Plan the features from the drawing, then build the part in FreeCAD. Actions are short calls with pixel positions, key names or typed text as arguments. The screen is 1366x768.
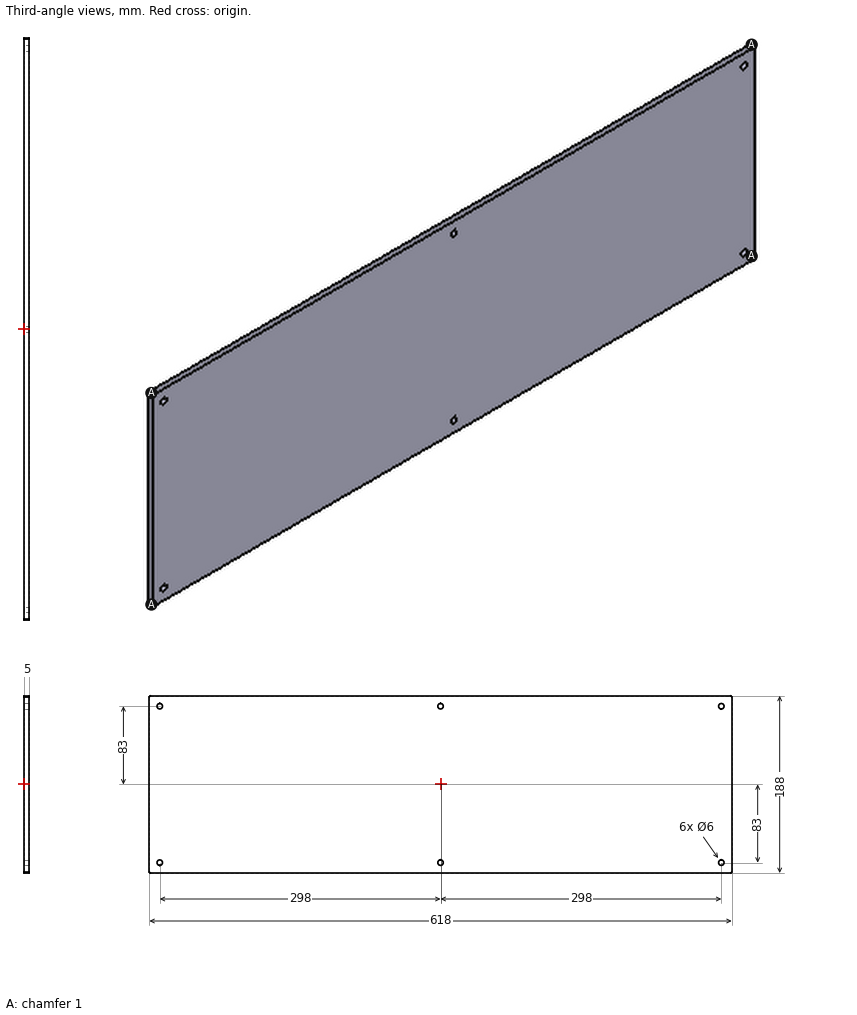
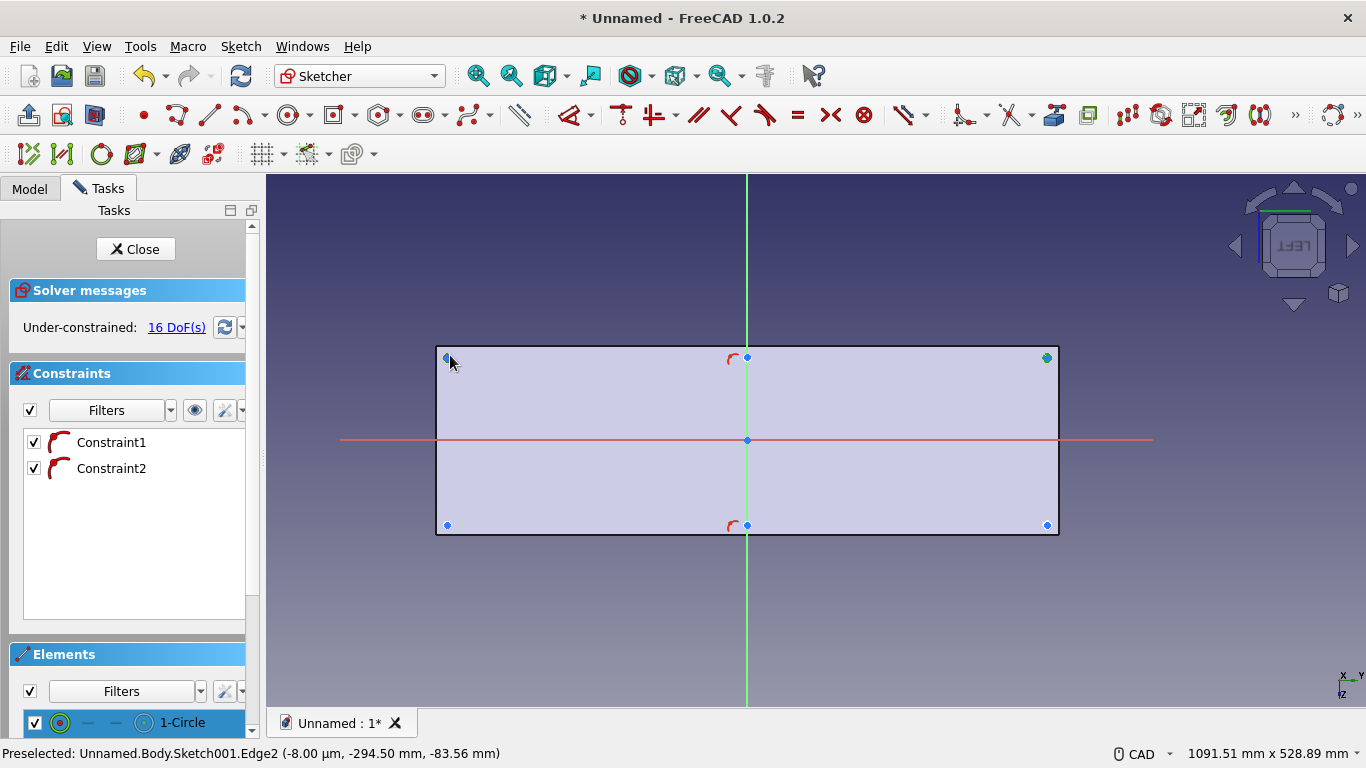
scroll(450, 523, up, 7)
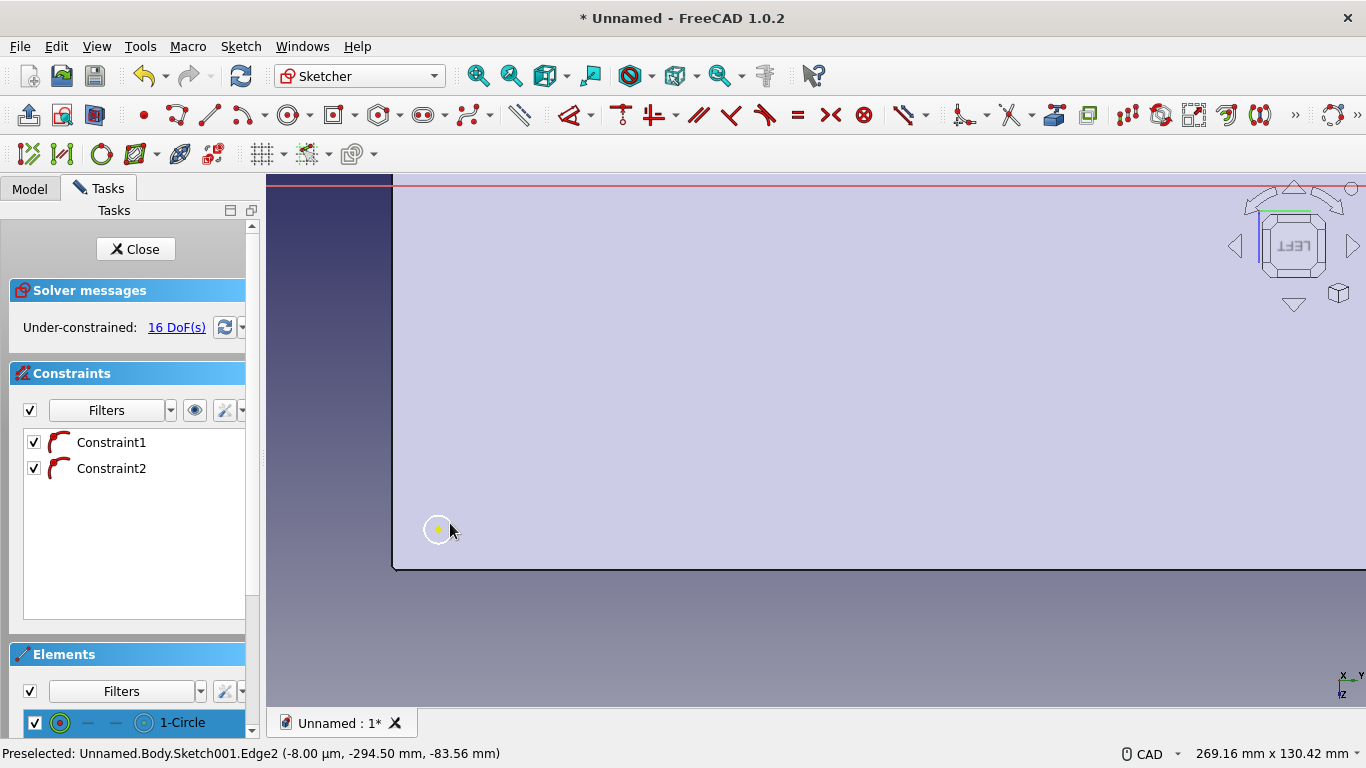
click(448, 520)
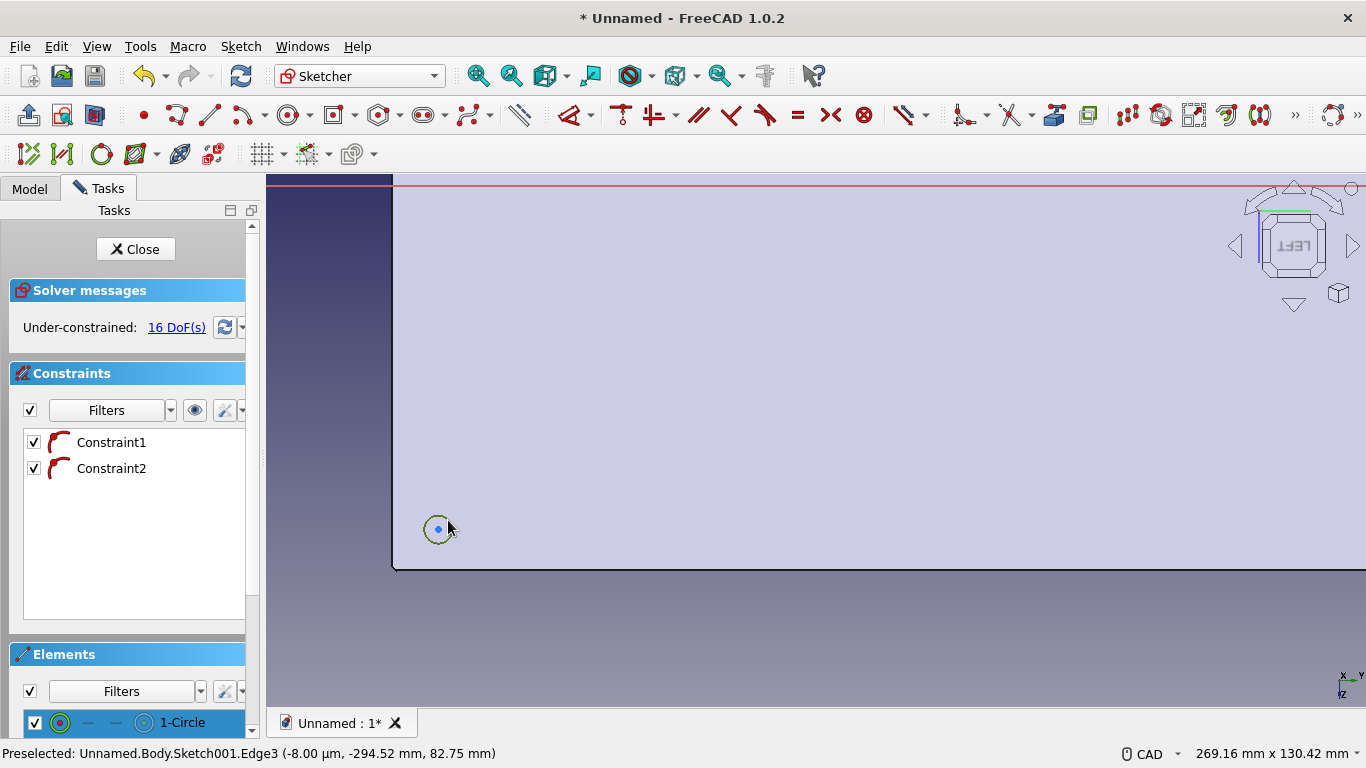
scroll(450, 524, down, 7)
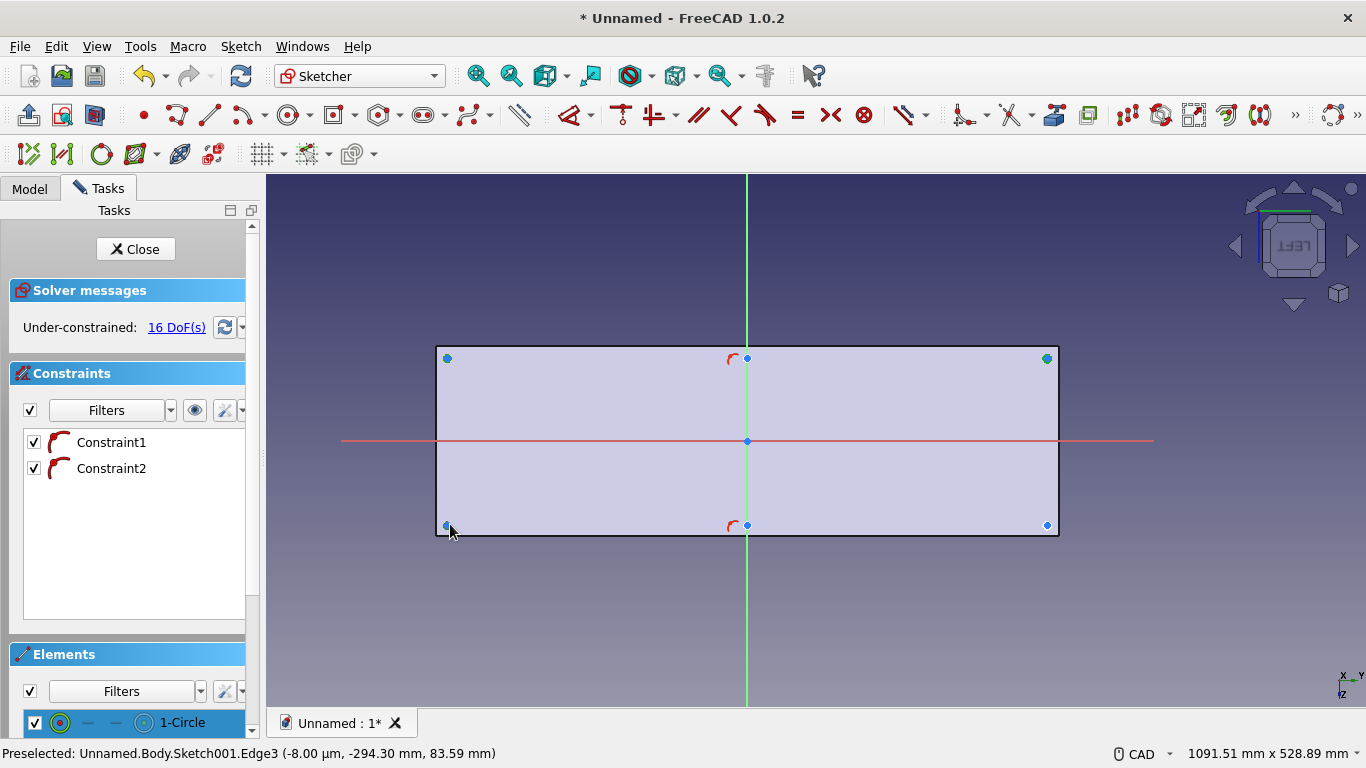
scroll(1050, 523, up, 7)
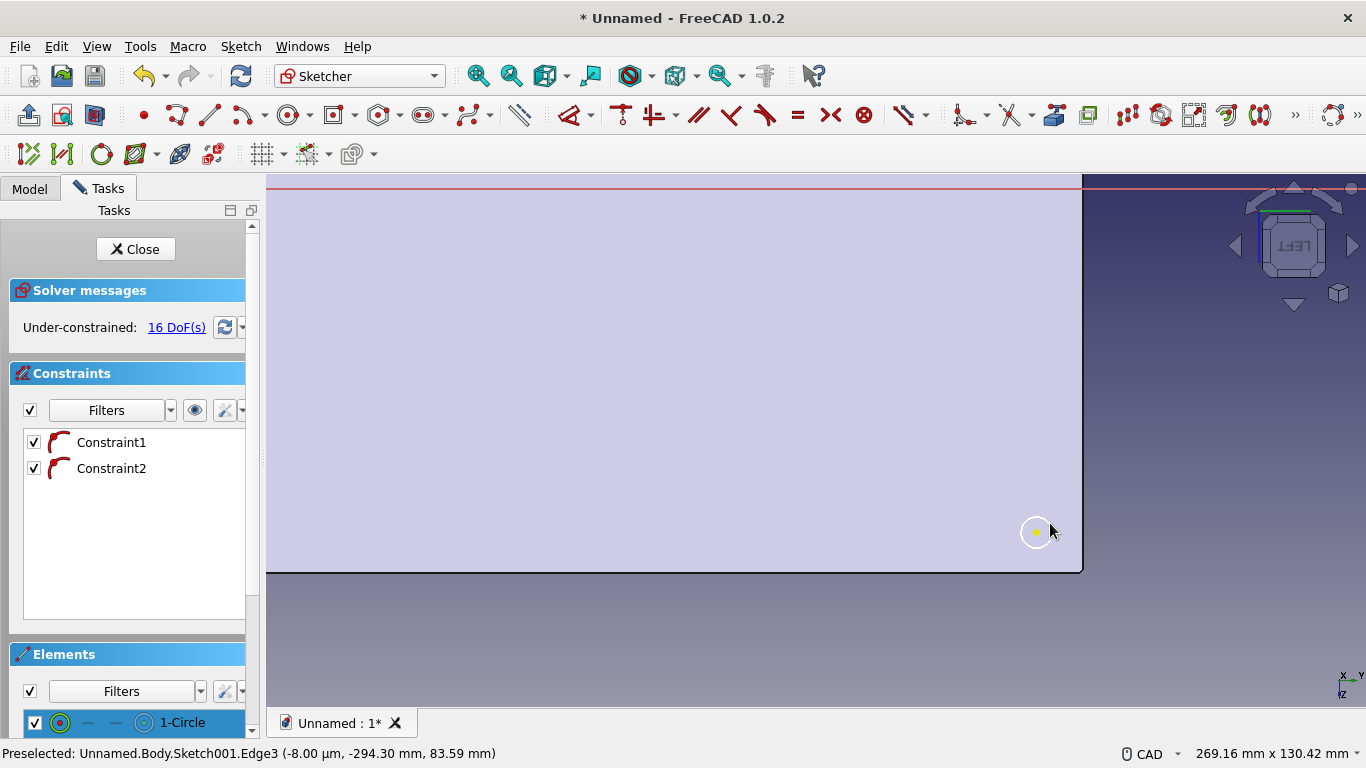
click(1048, 522)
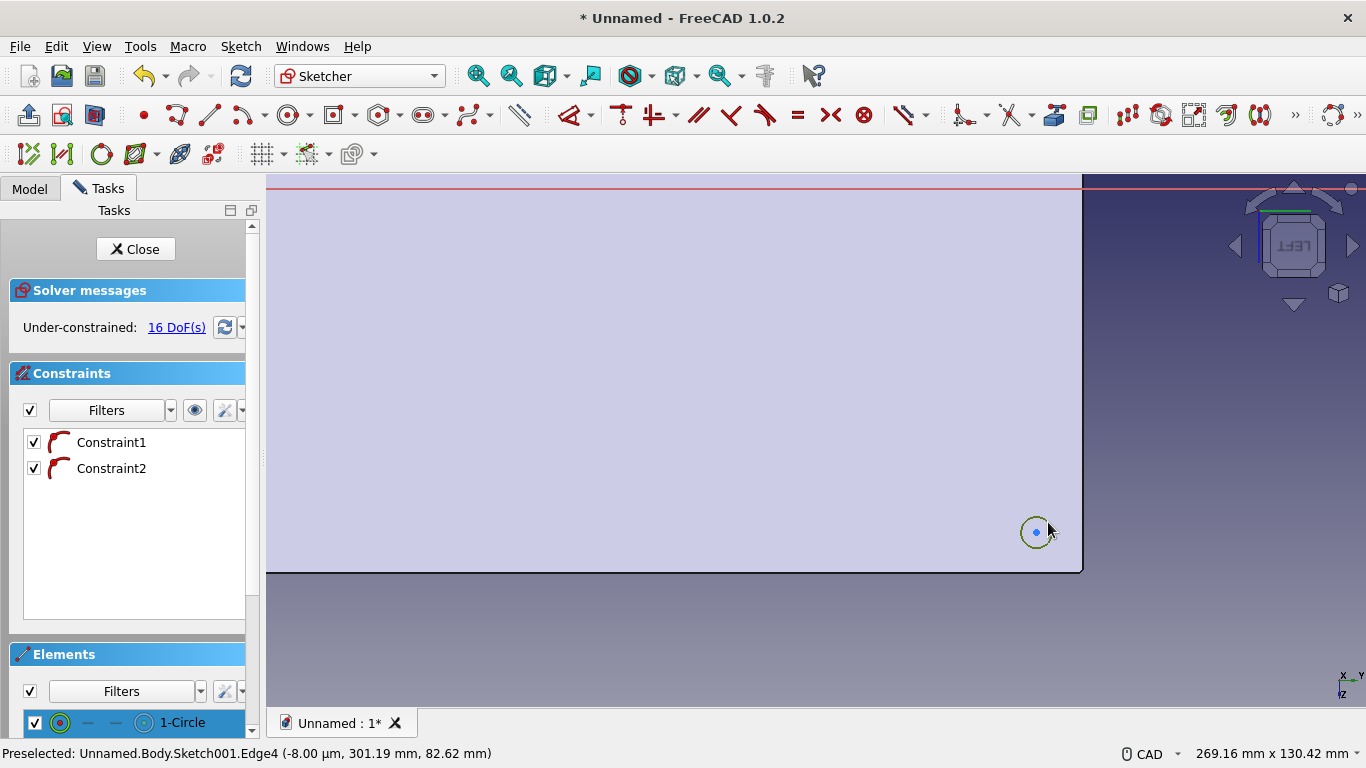
scroll(1051, 523, down, 7)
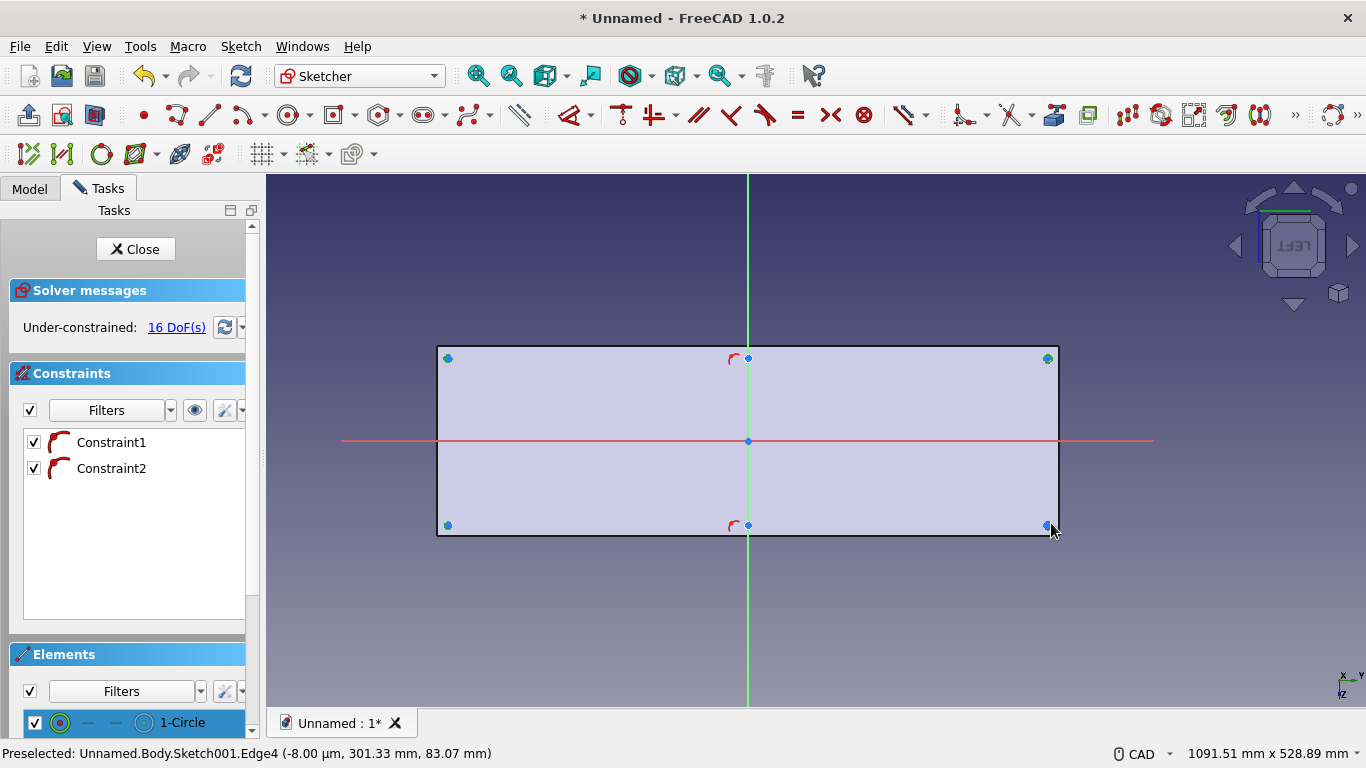
scroll(750, 523, up, 9)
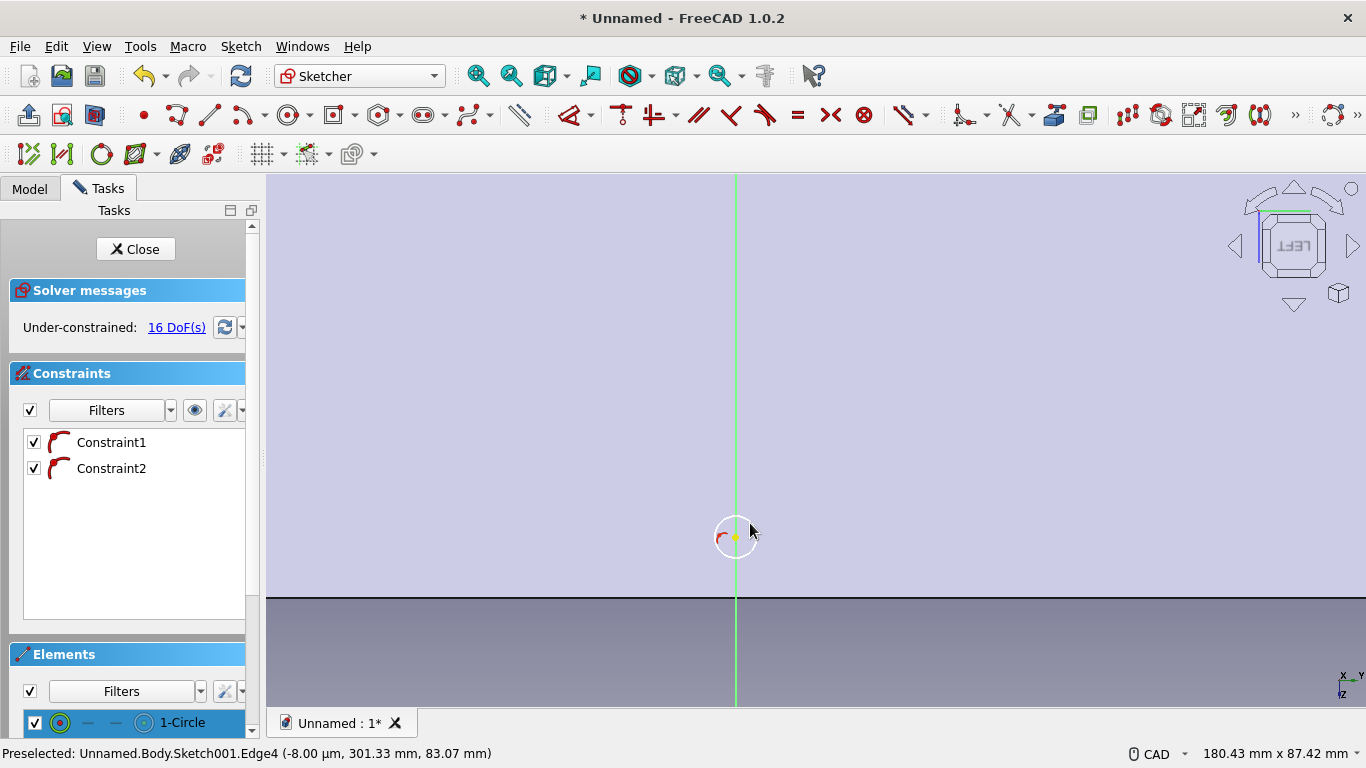
click(751, 522)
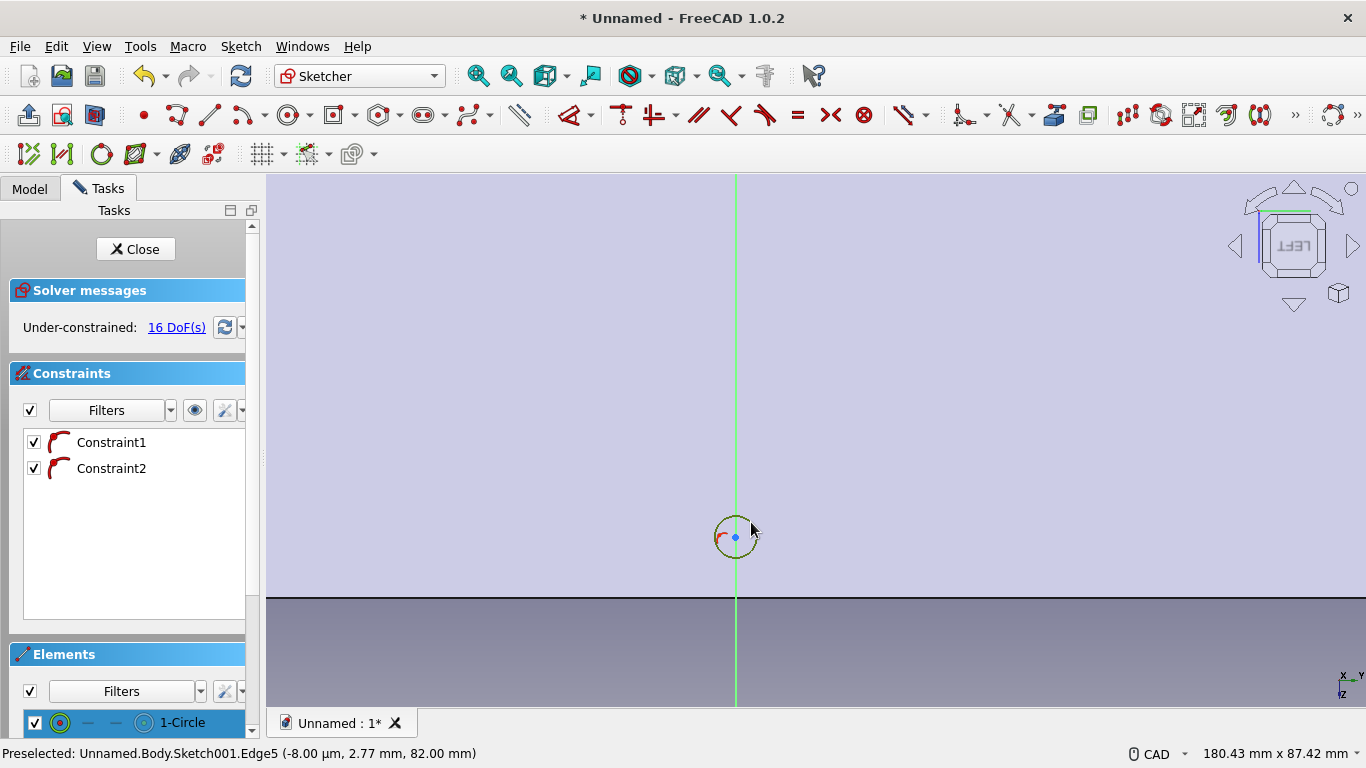
scroll(750, 523, down, 9)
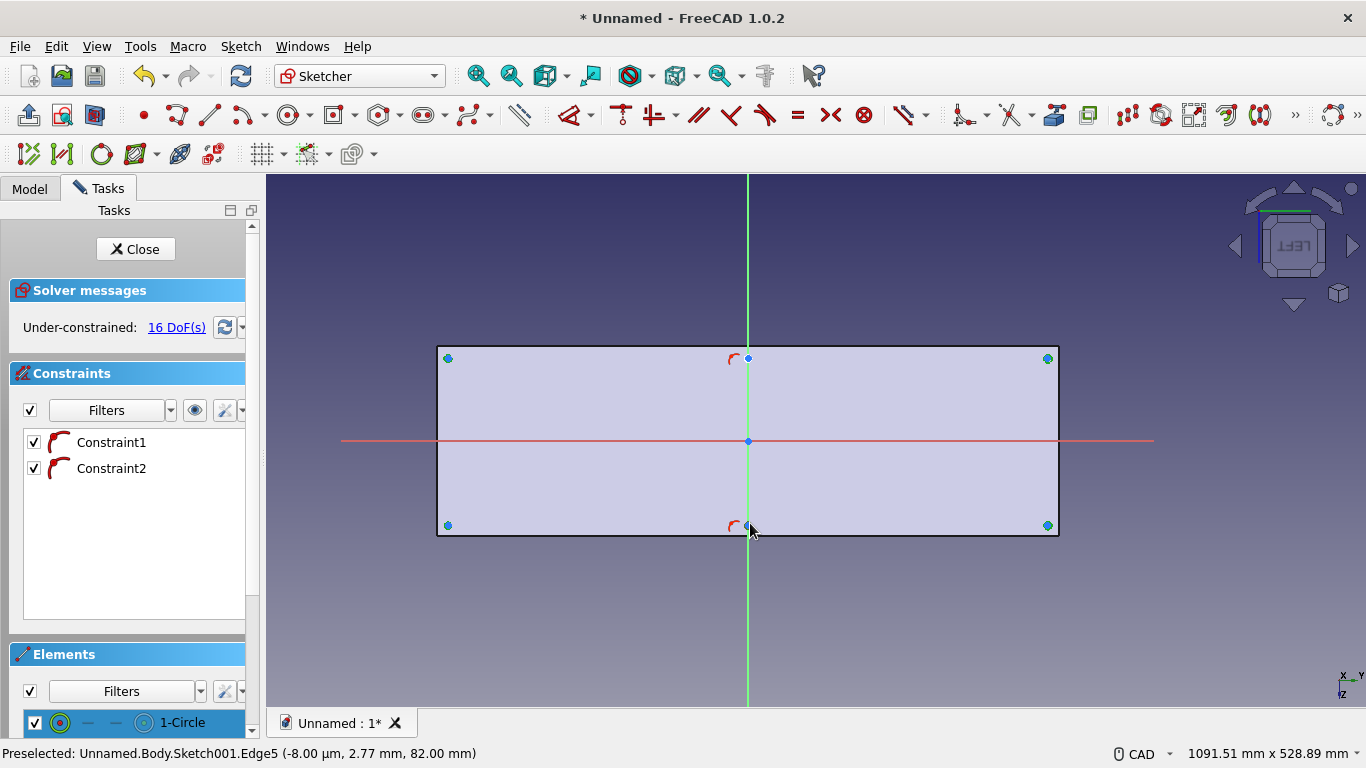
scroll(750, 356, up, 9)